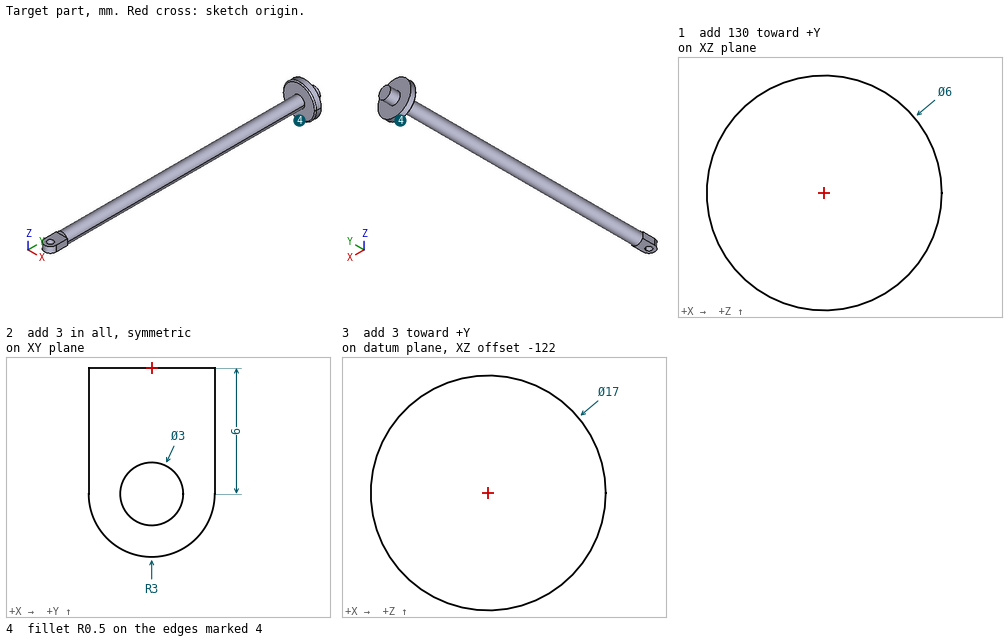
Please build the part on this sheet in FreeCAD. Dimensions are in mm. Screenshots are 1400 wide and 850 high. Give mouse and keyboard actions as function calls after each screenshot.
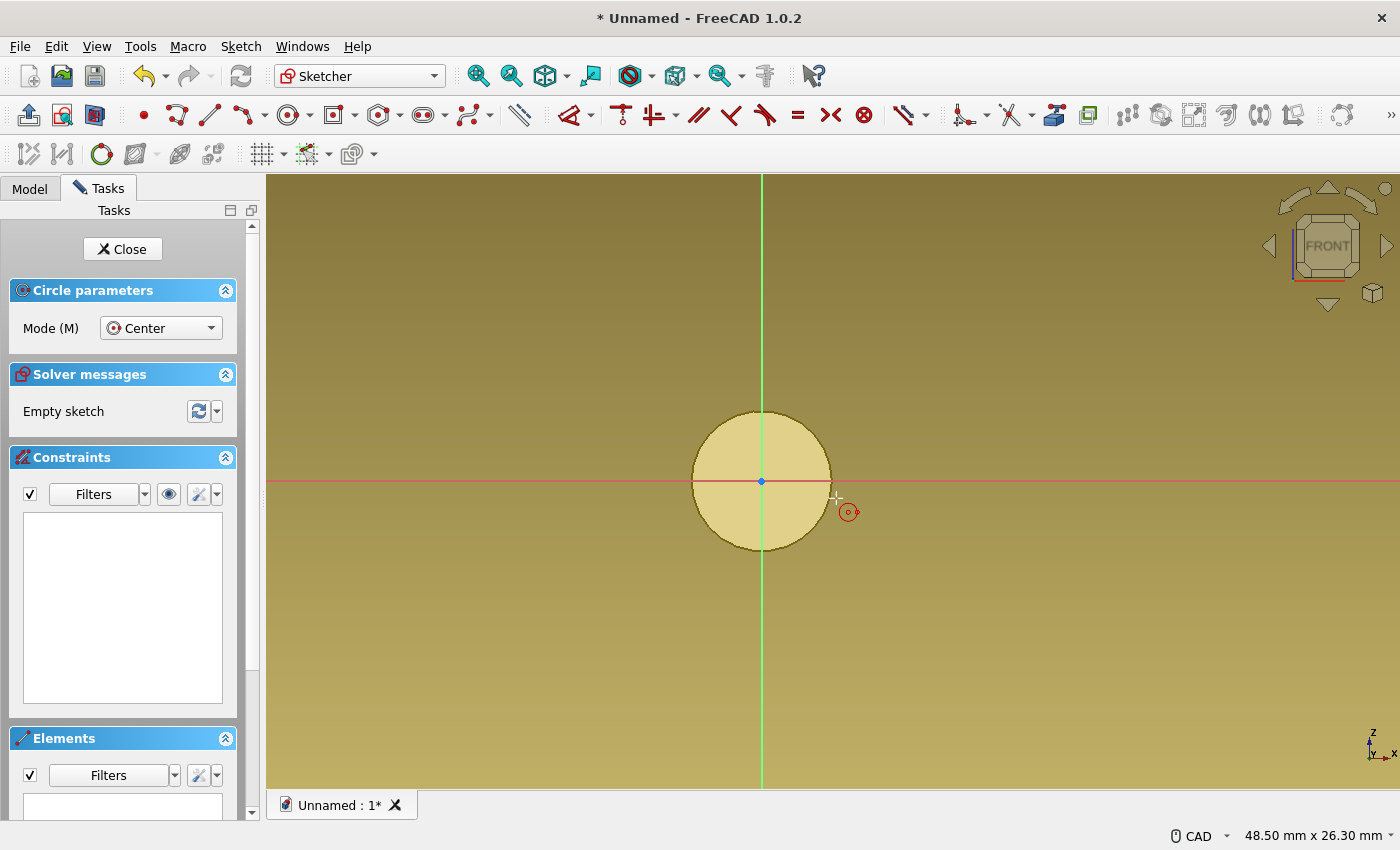
click(762, 481)
click(902, 341)
key(Escape)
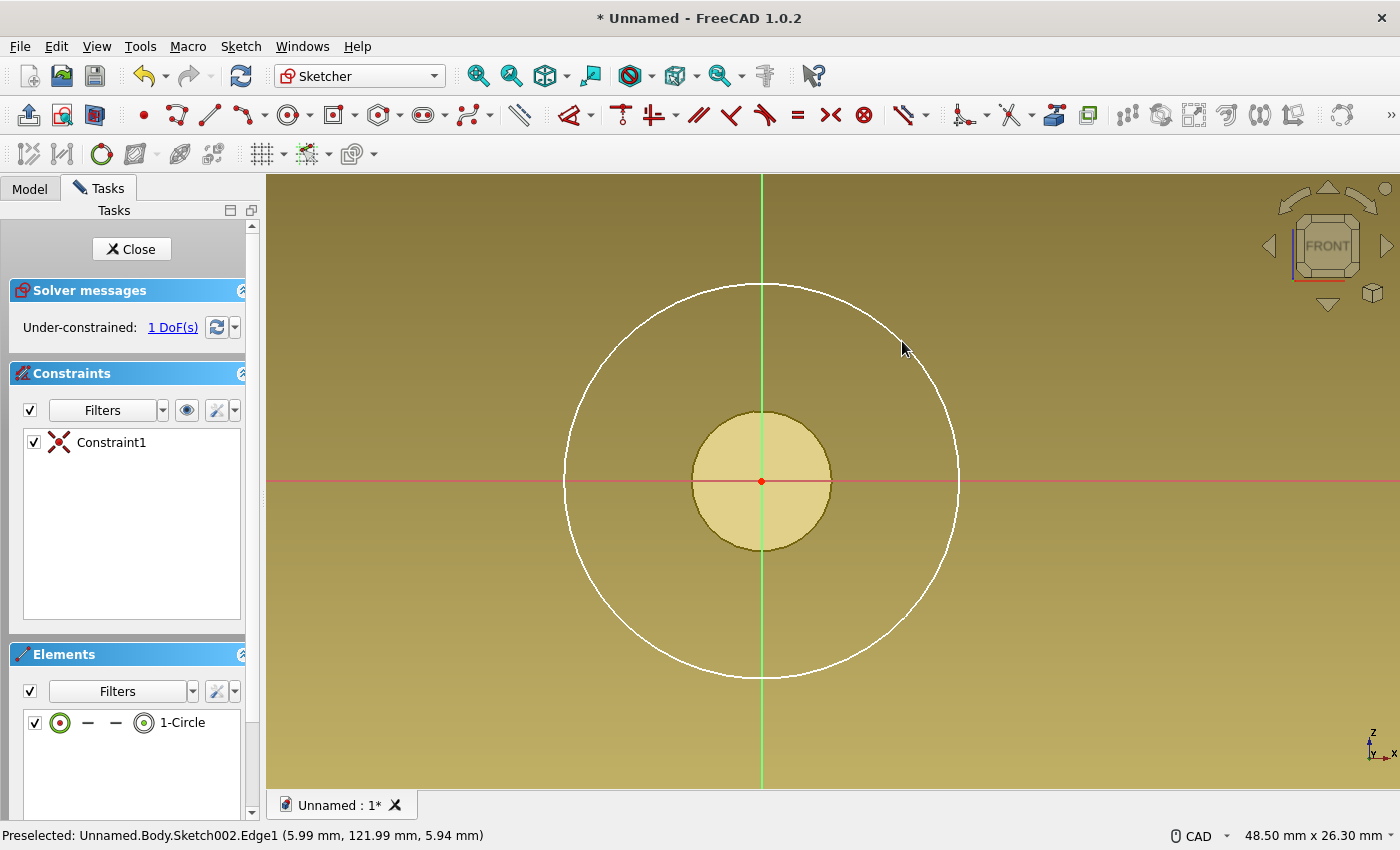
key(d)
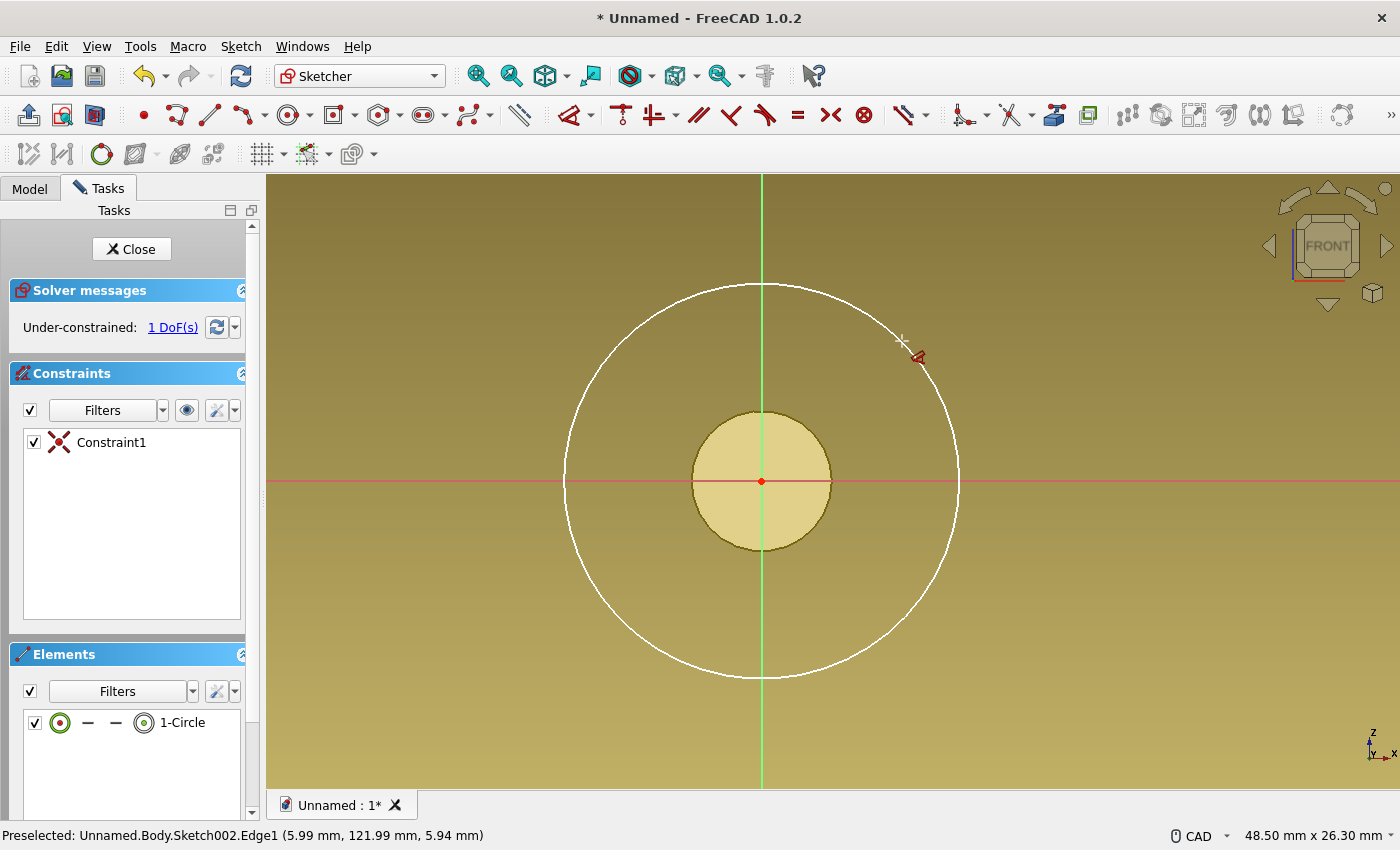
click(901, 341)
click(924, 318)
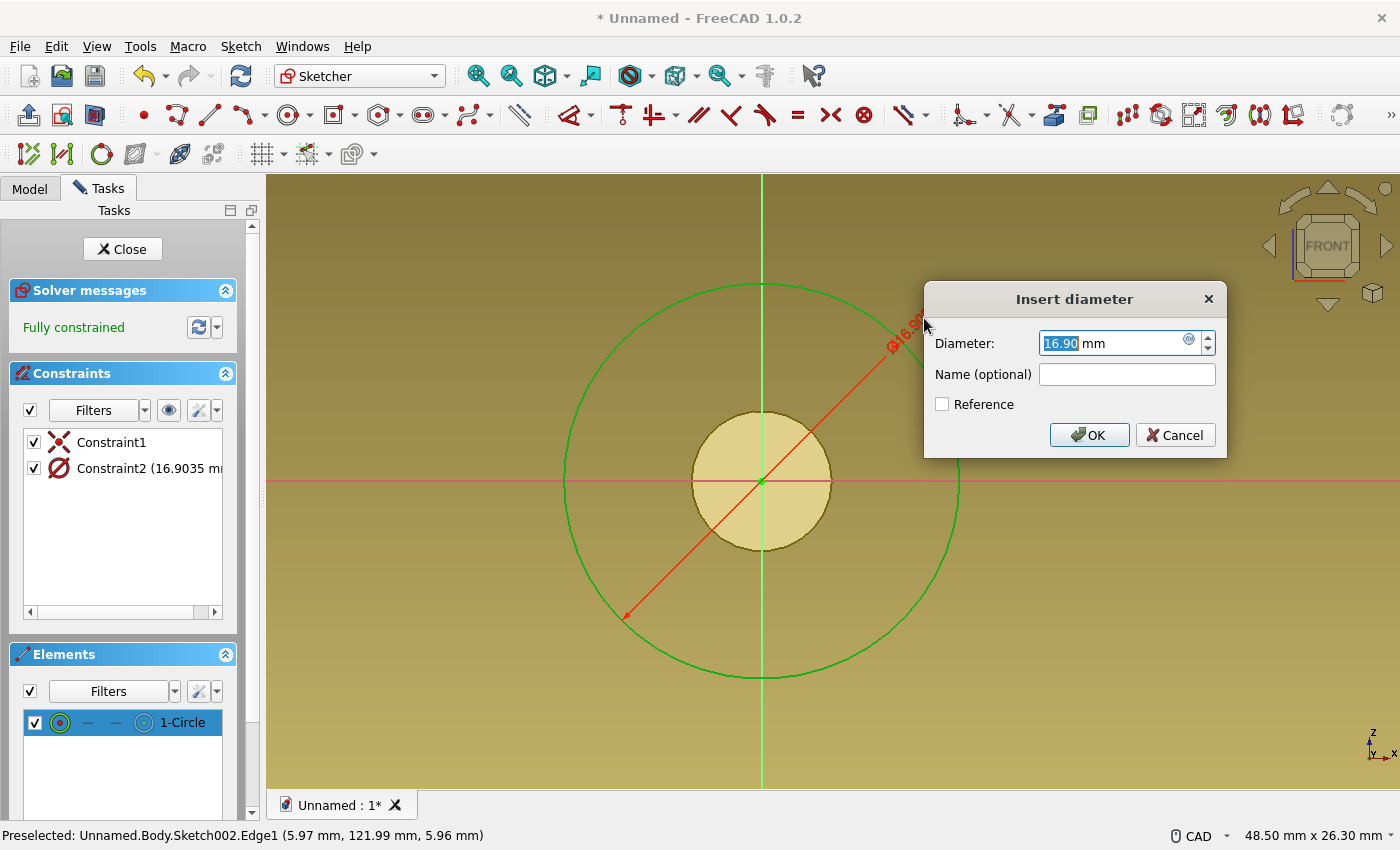
text(17)
key(Return)
key(Escape)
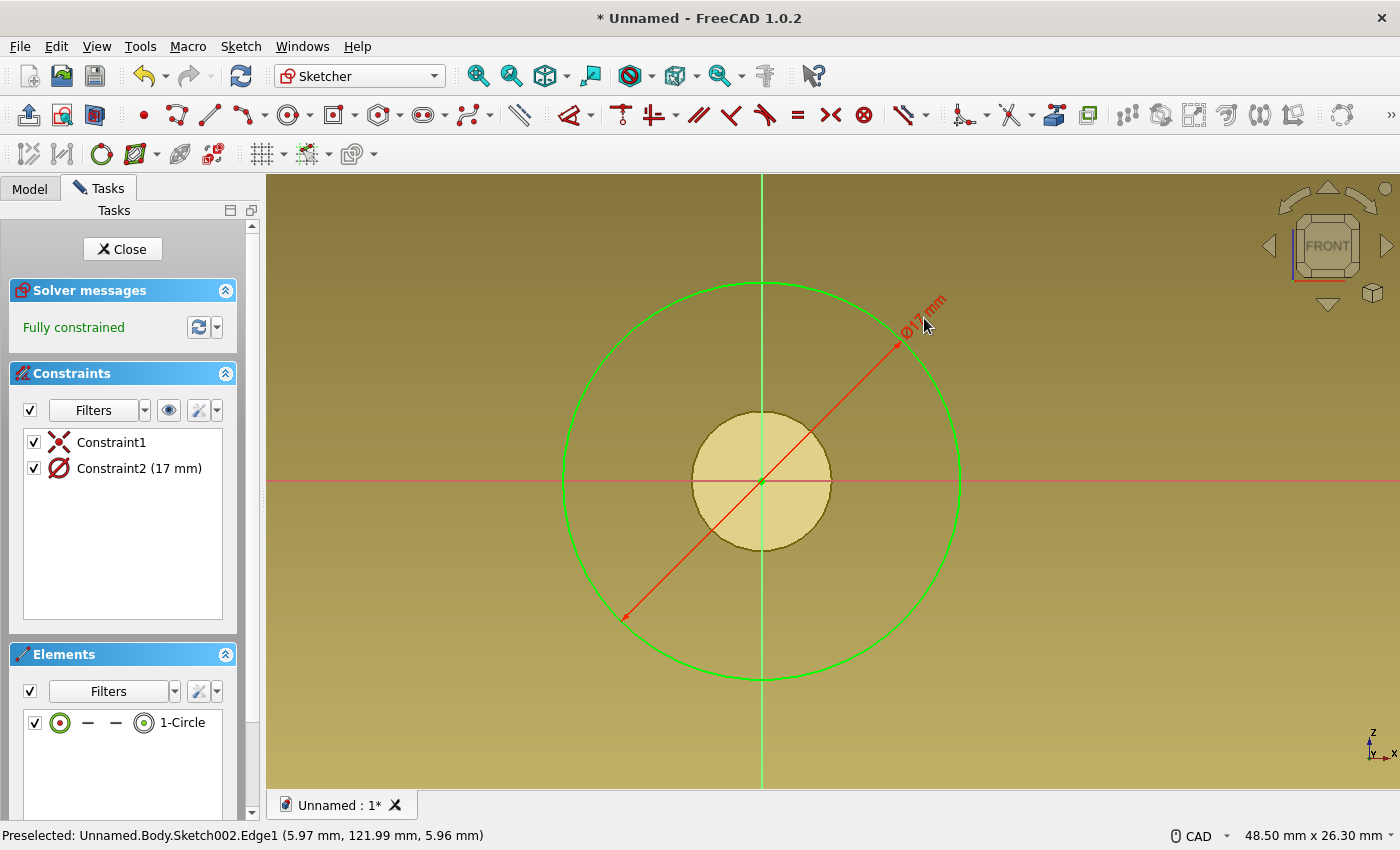
click(123, 249)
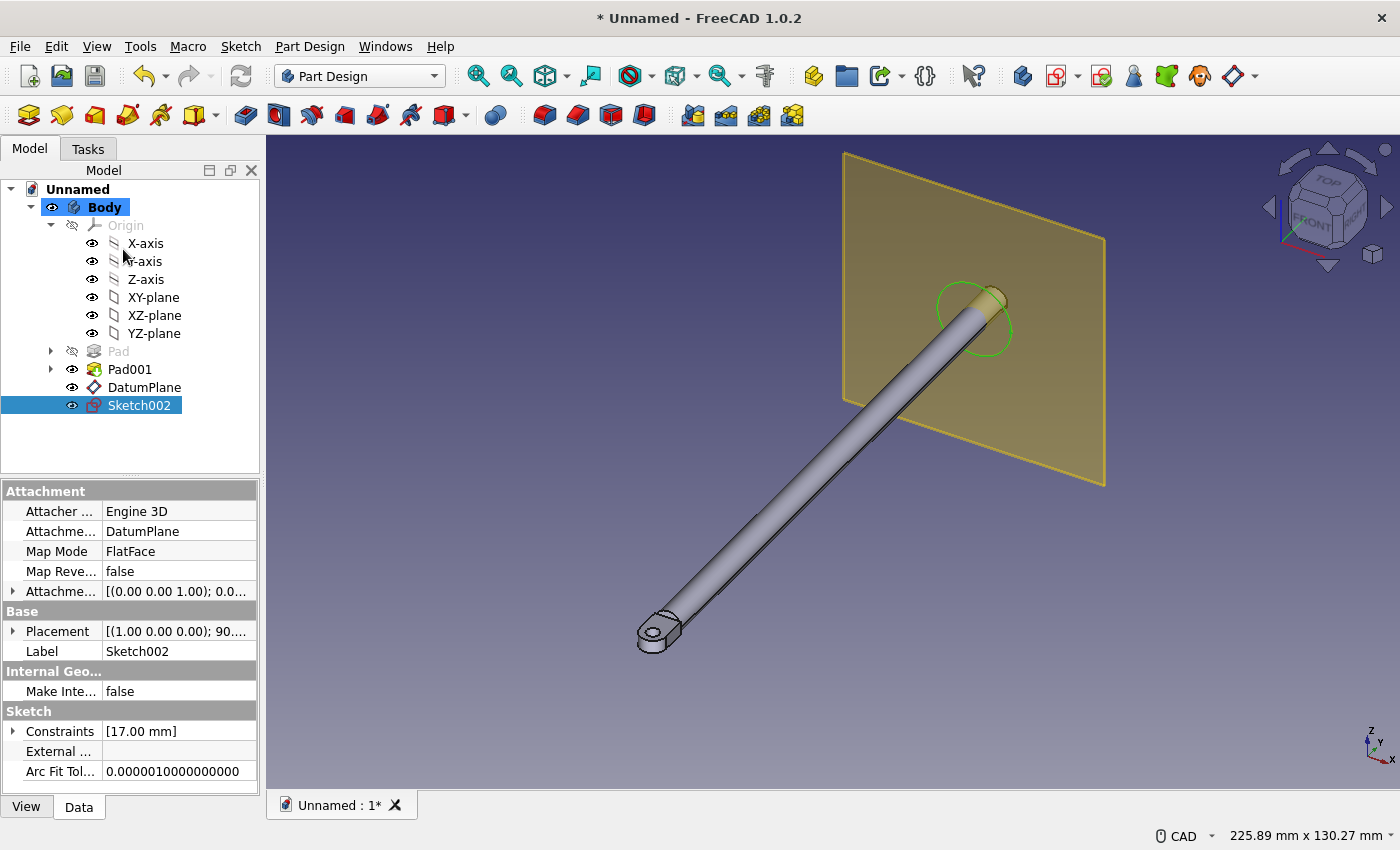
click(29, 116)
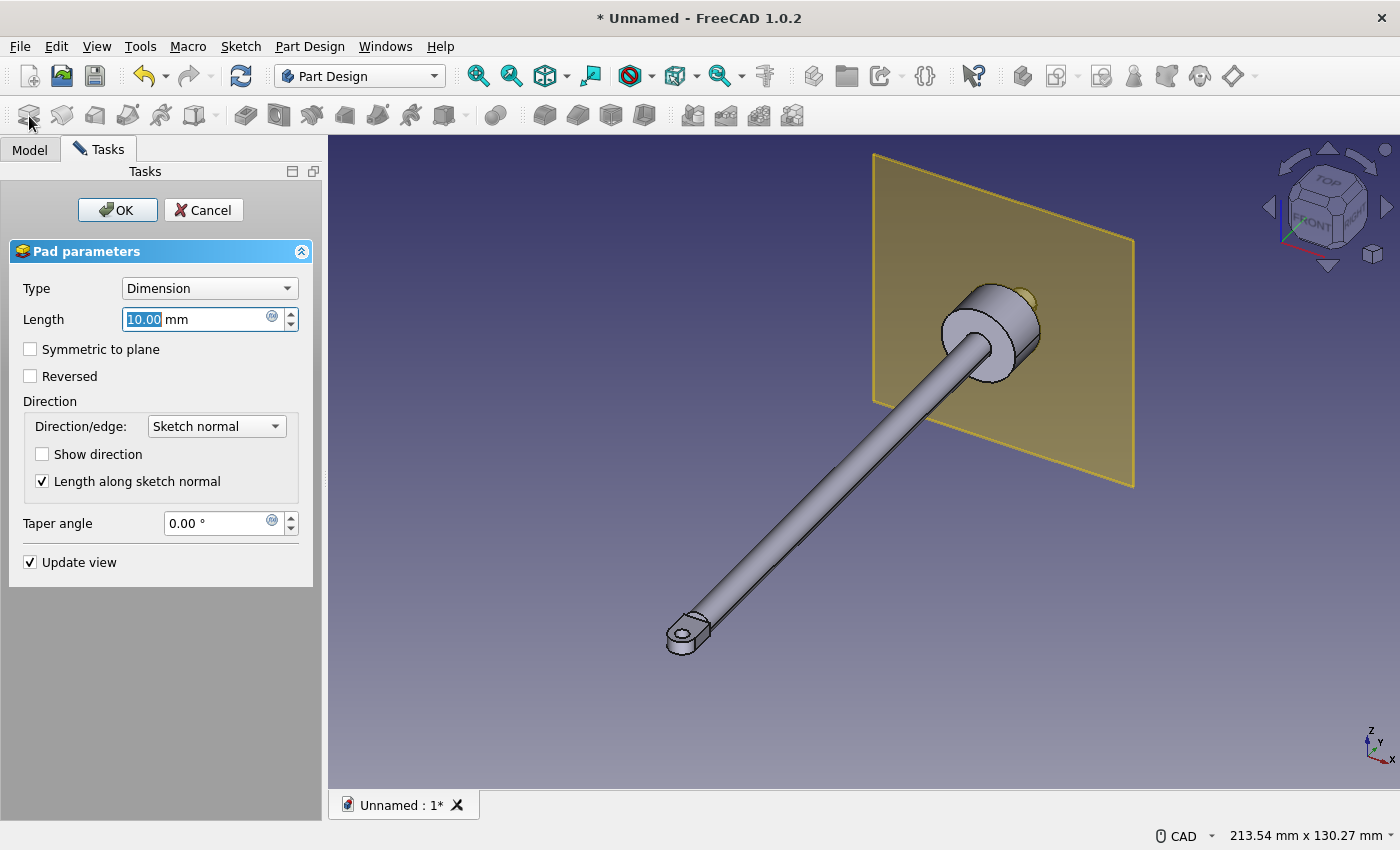
text(3)
key(Tab)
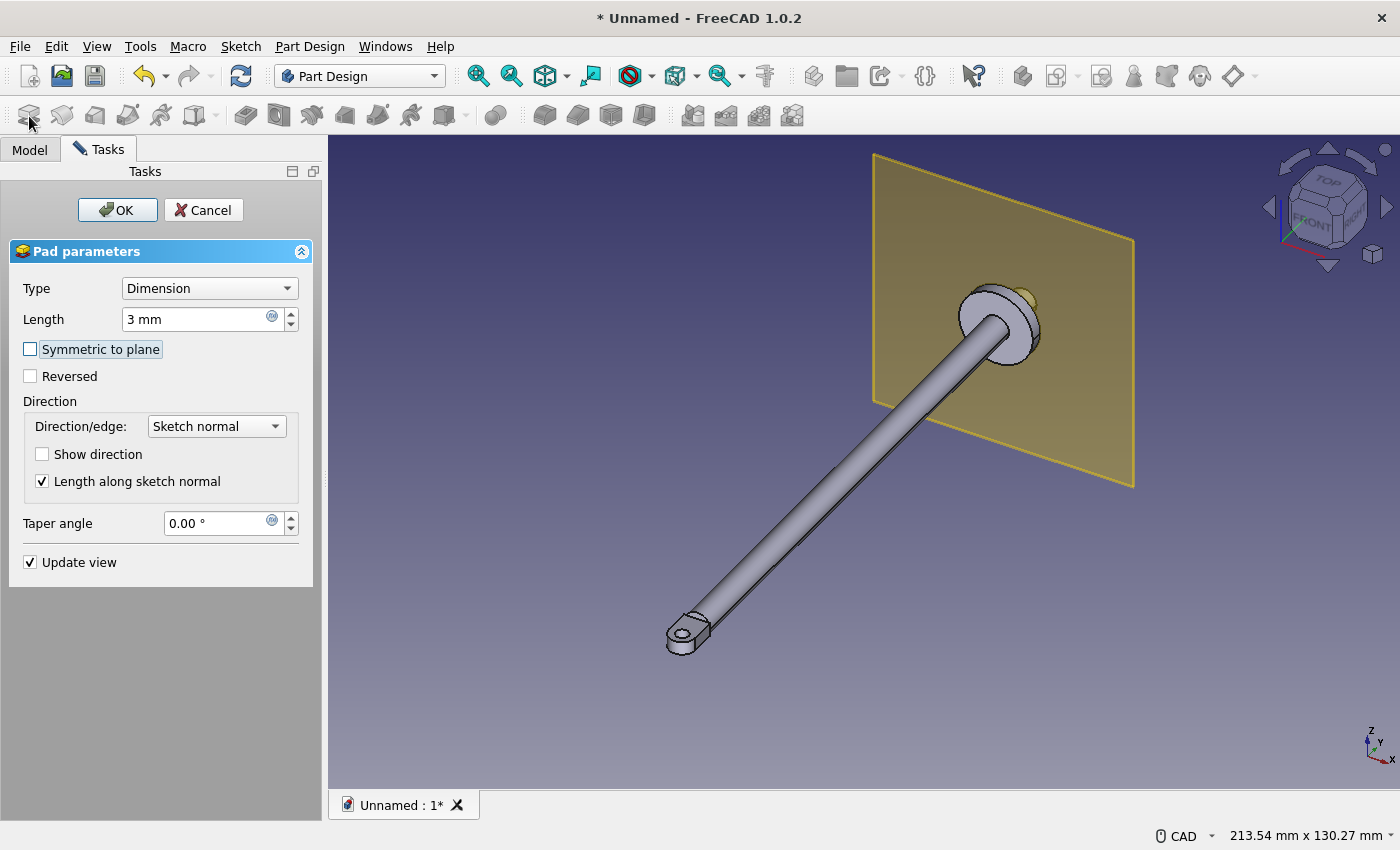
click(31, 376)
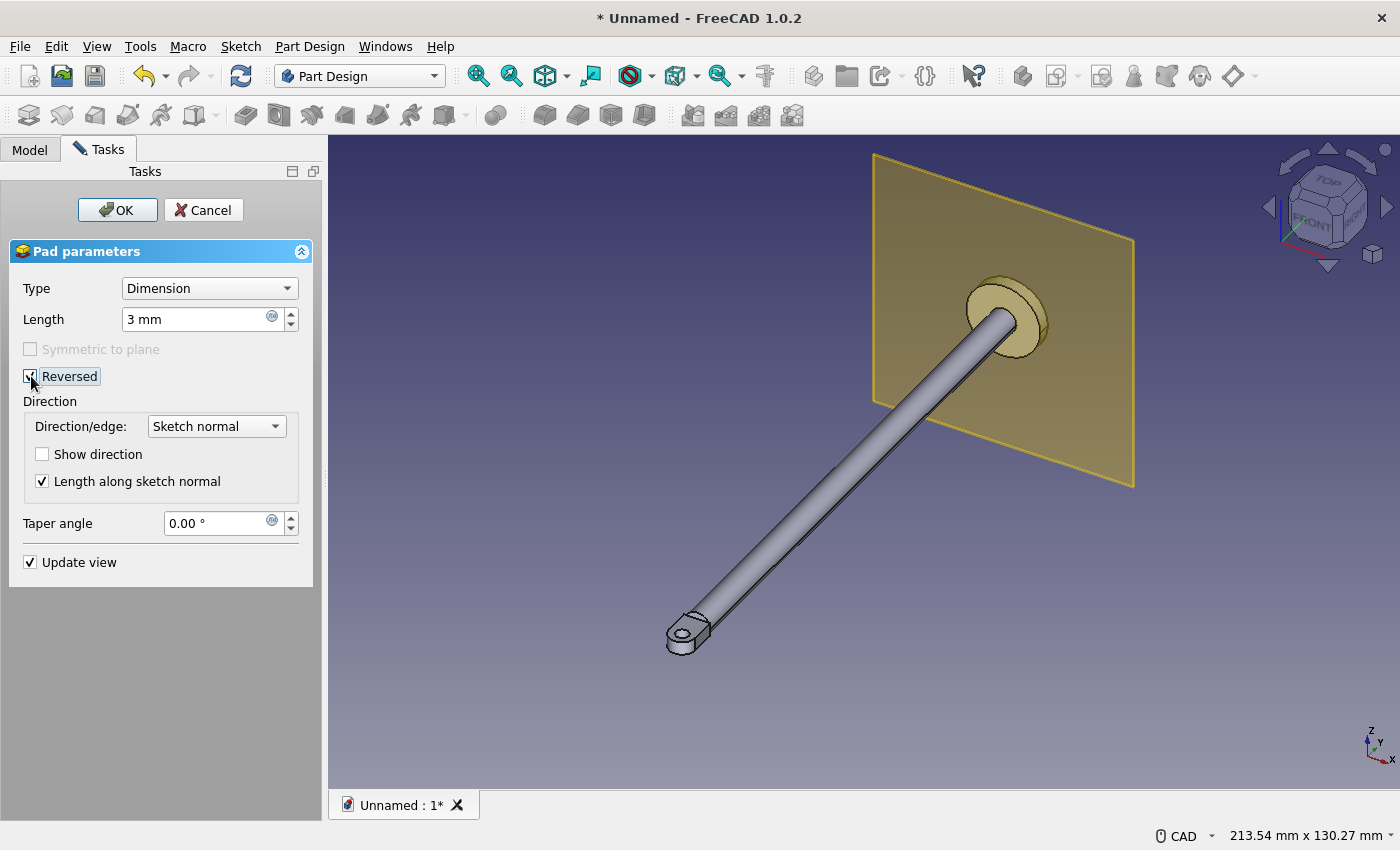
click(118, 210)